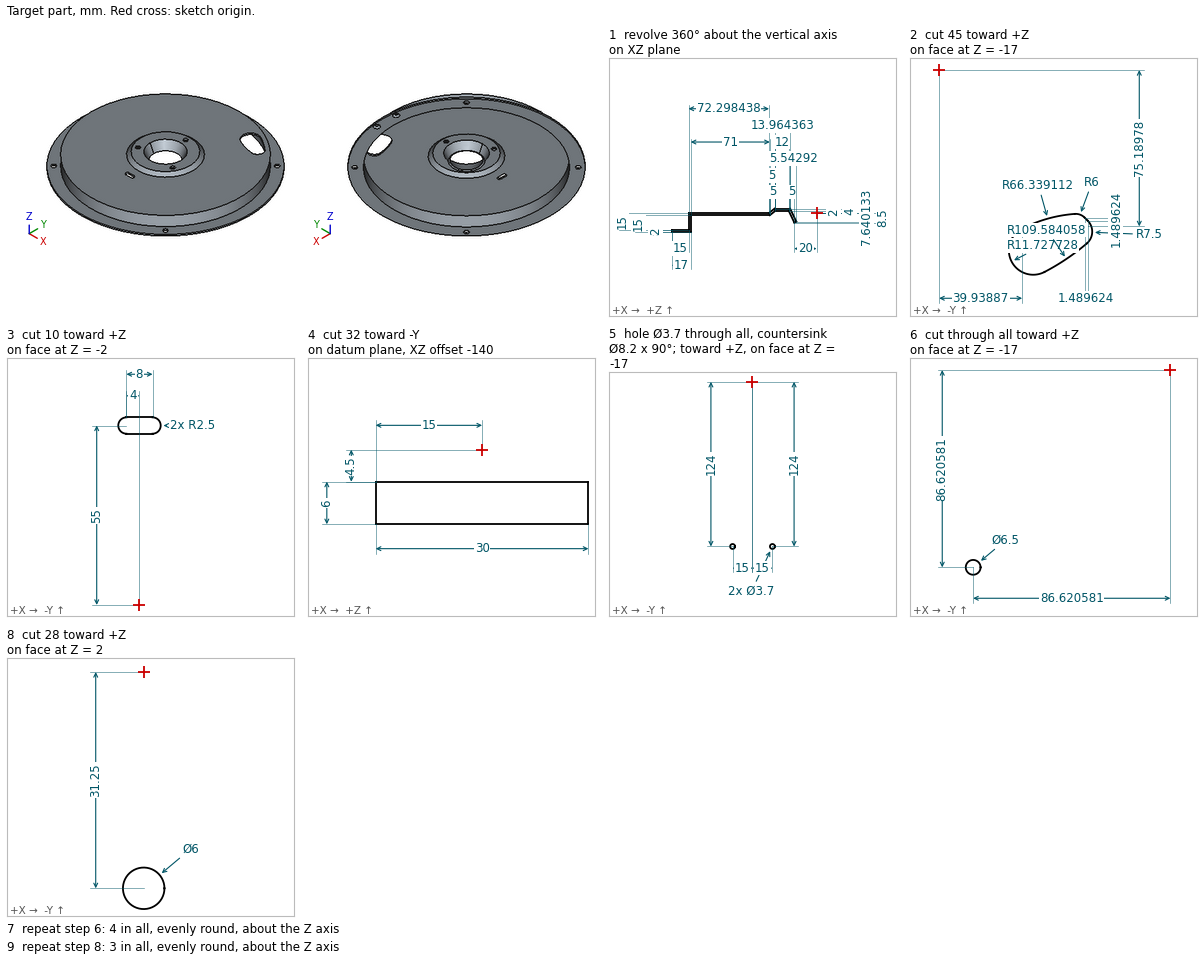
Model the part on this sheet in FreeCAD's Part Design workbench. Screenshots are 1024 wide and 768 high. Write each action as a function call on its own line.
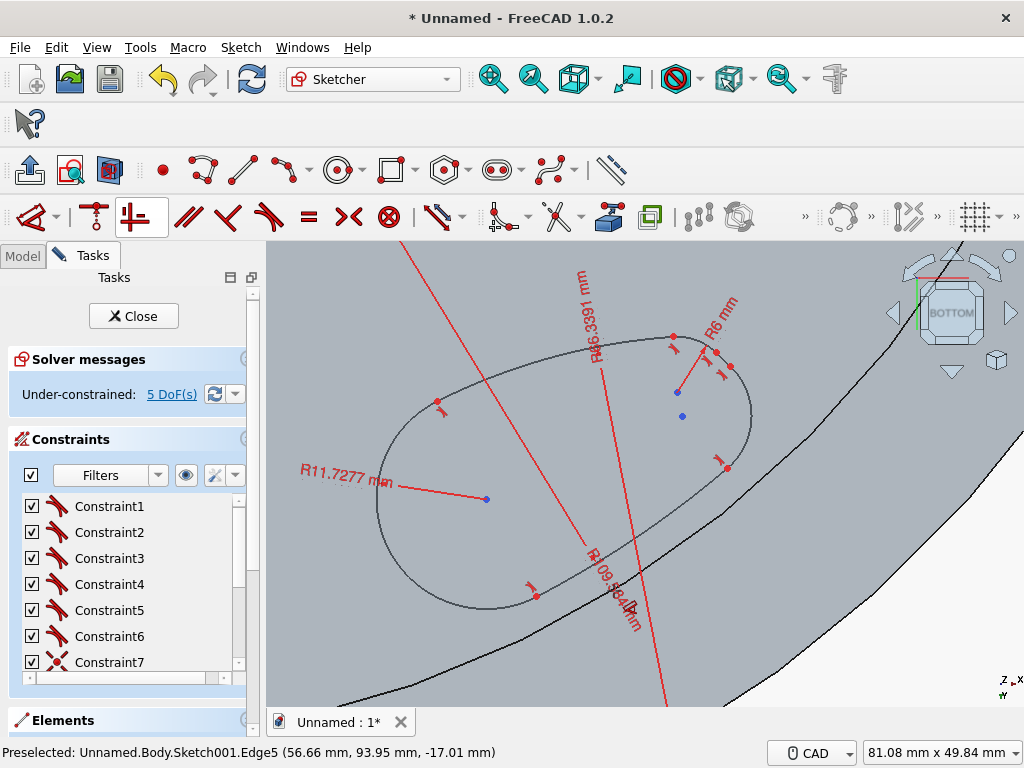
click(747, 441)
click(777, 453)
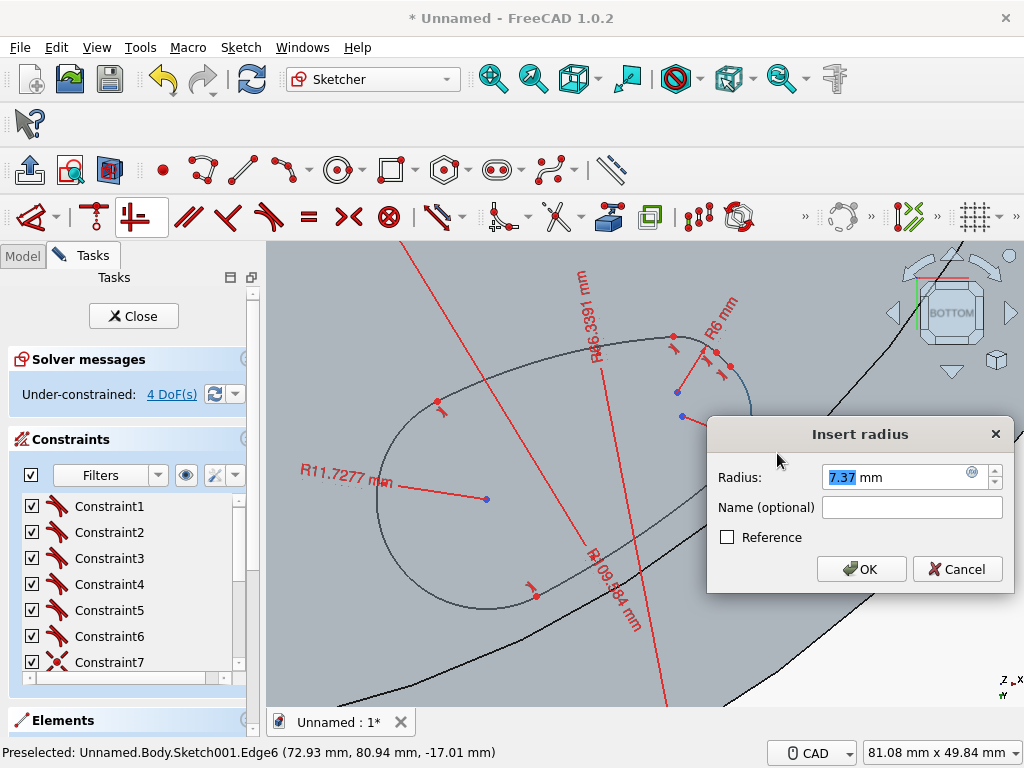
text(7.5)
key(Return)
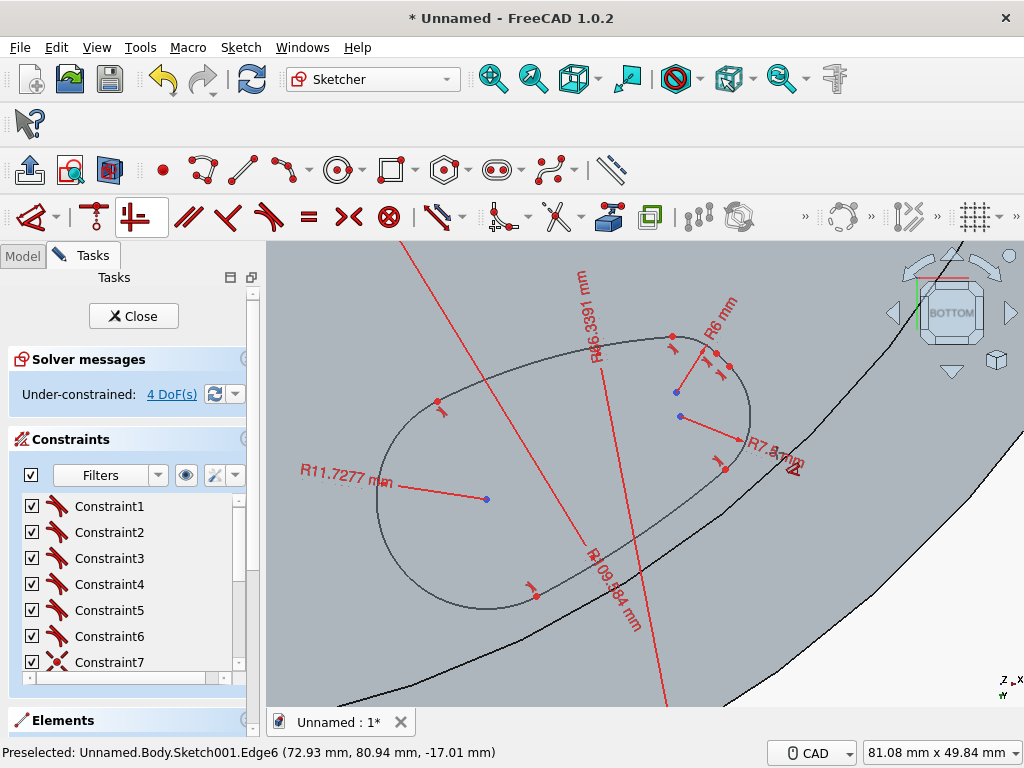
click(437, 401)
click(366, 435)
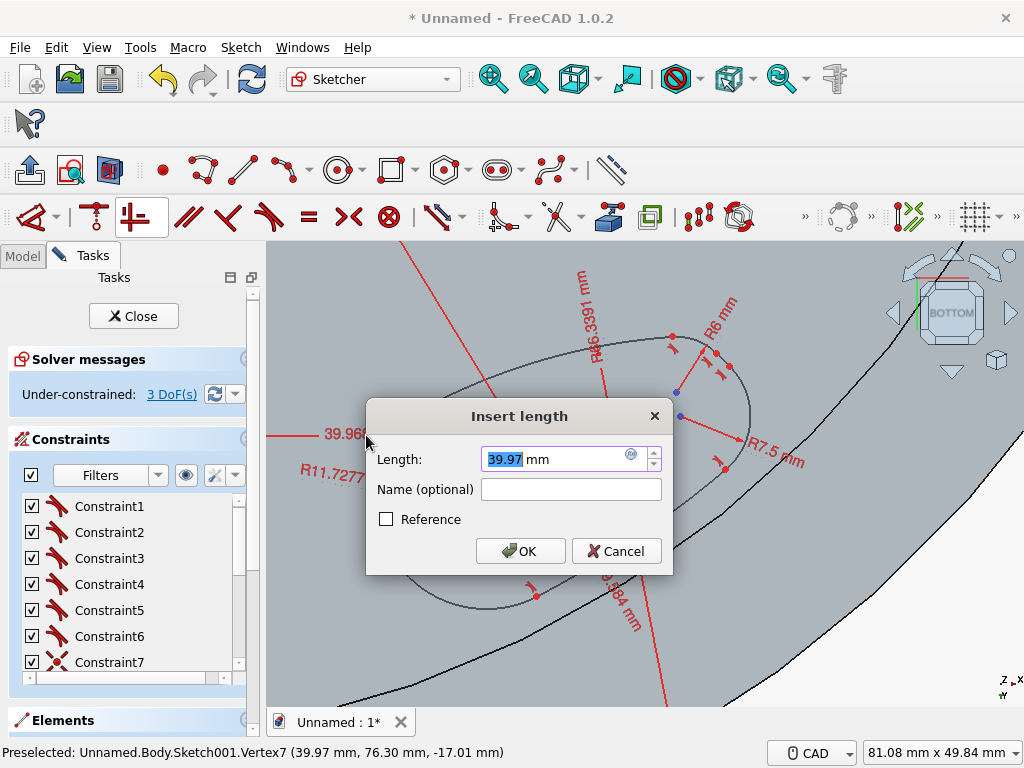
text(39.93887)
key(Return)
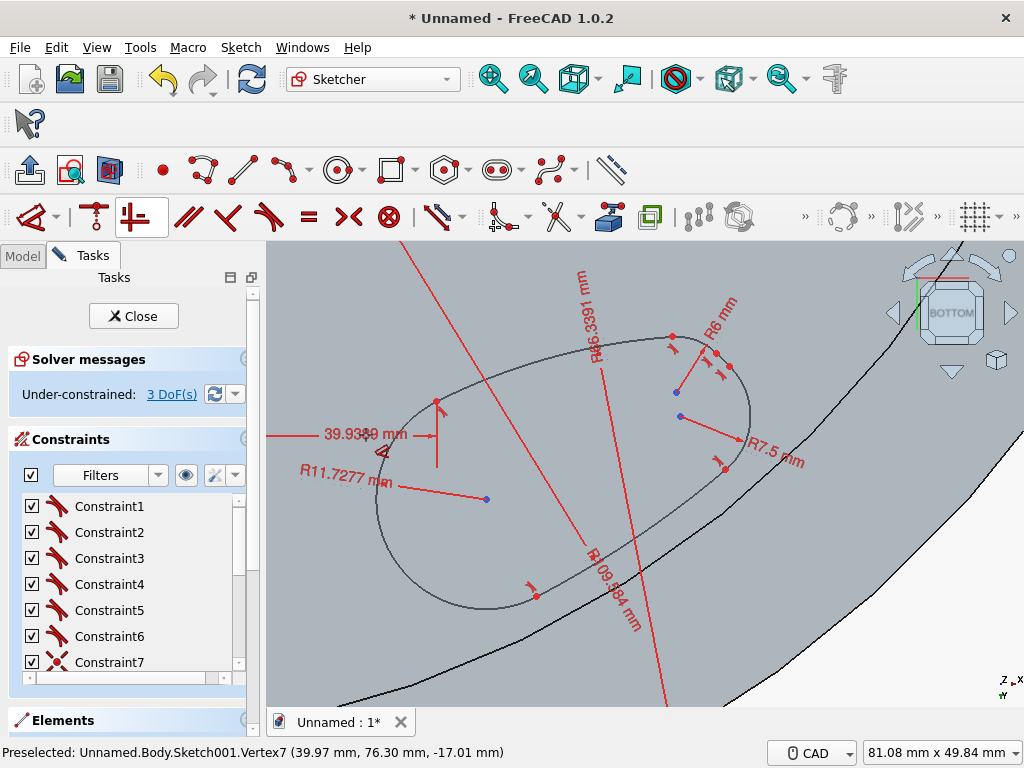
scroll(723, 360, up, 6)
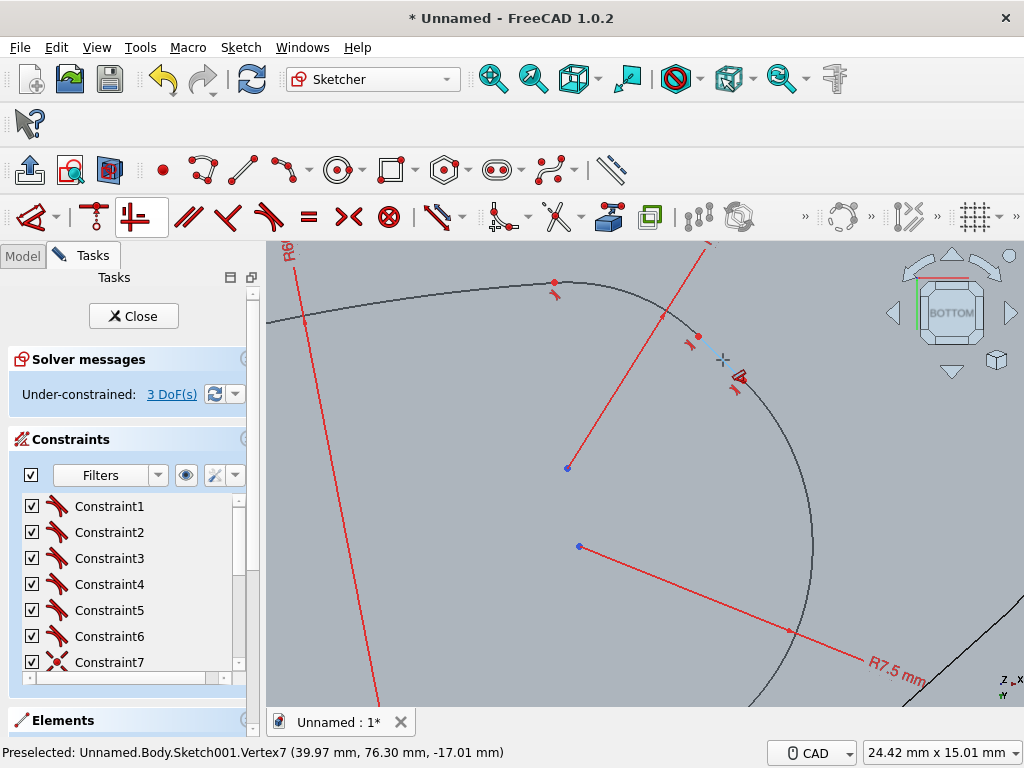
click(721, 359)
click(721, 302)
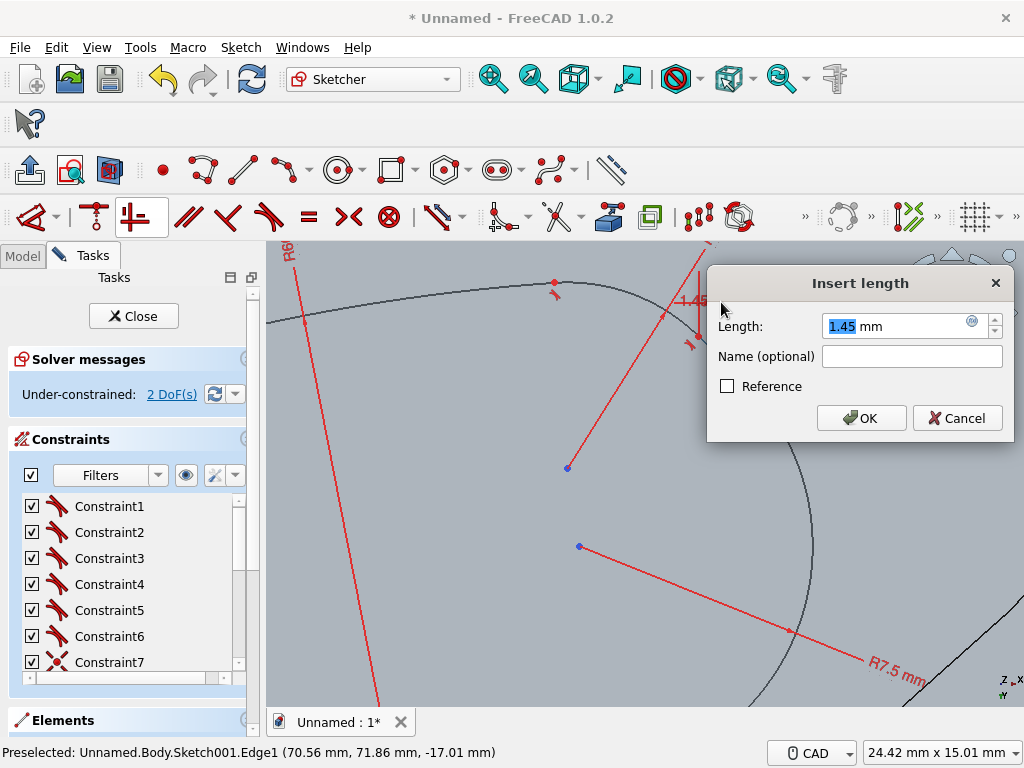
text(1.489624)
key(Return)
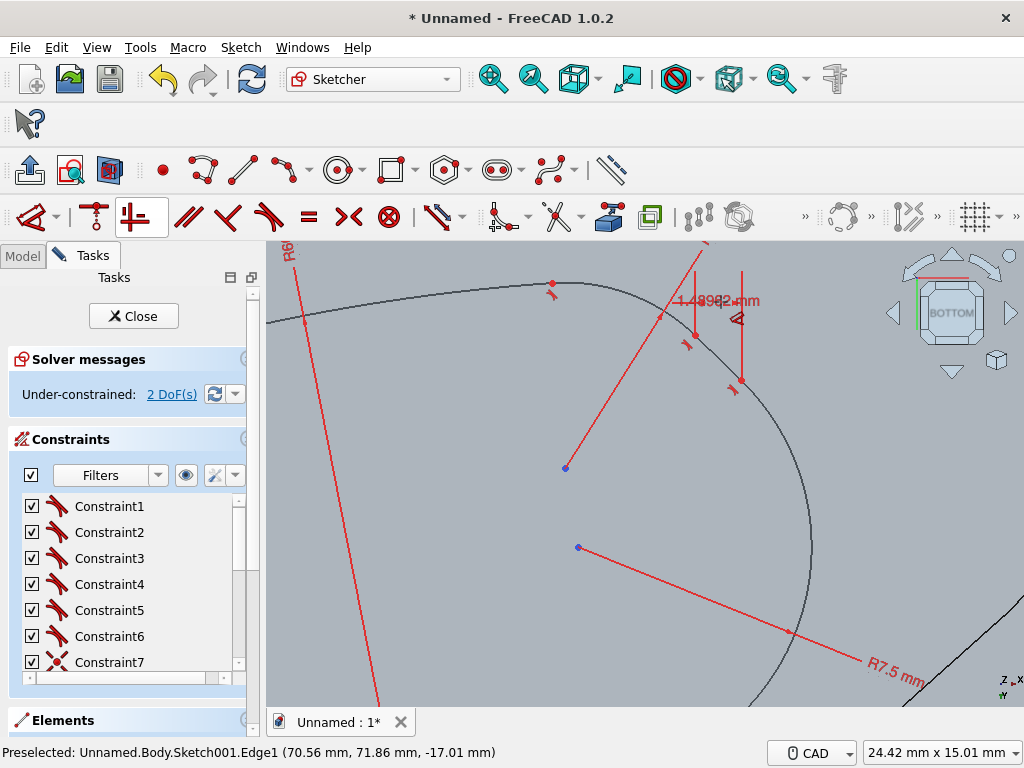
click(728, 367)
click(776, 358)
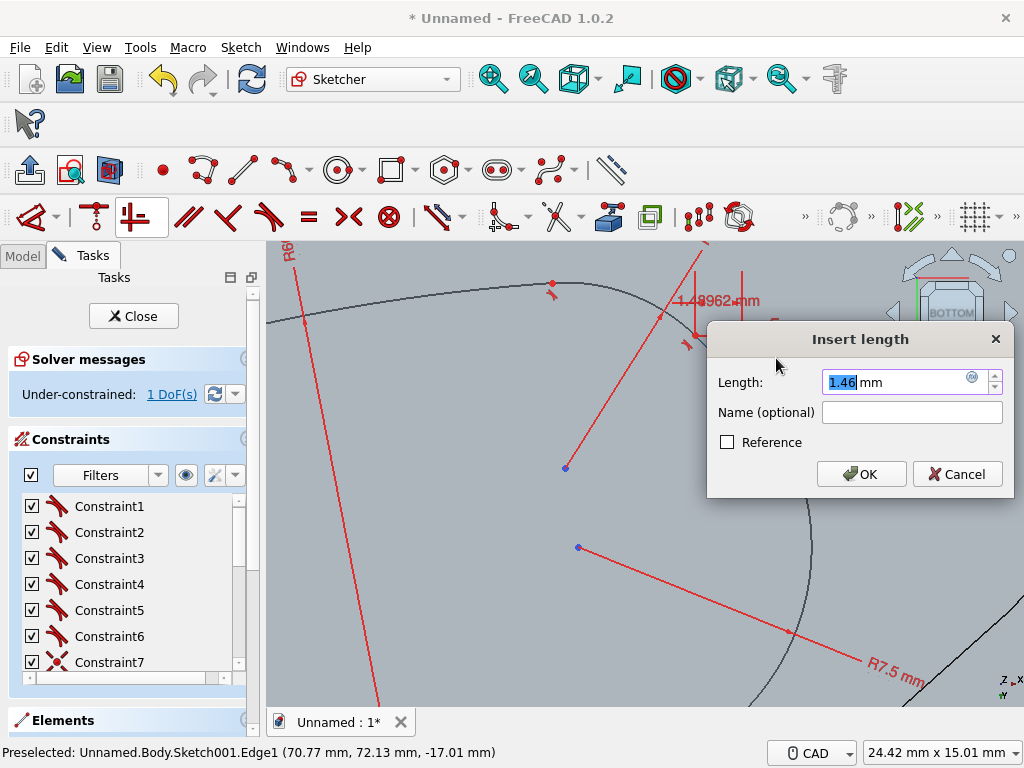
text(1.489624)
key(Return)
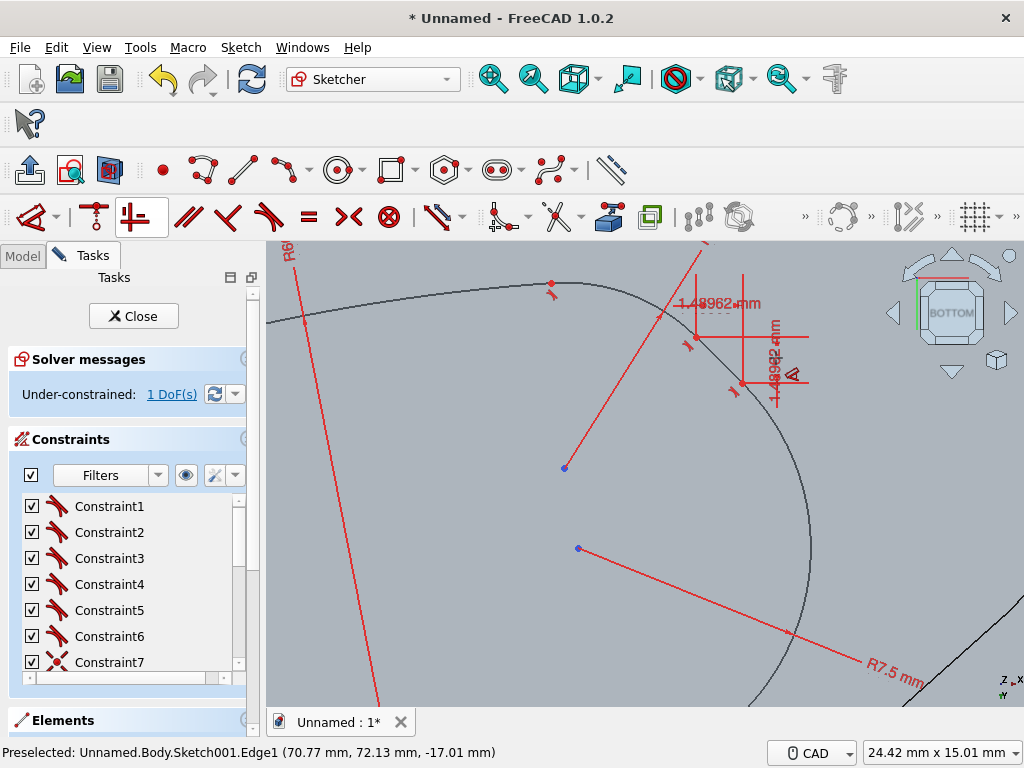
click(565, 469)
click(599, 369)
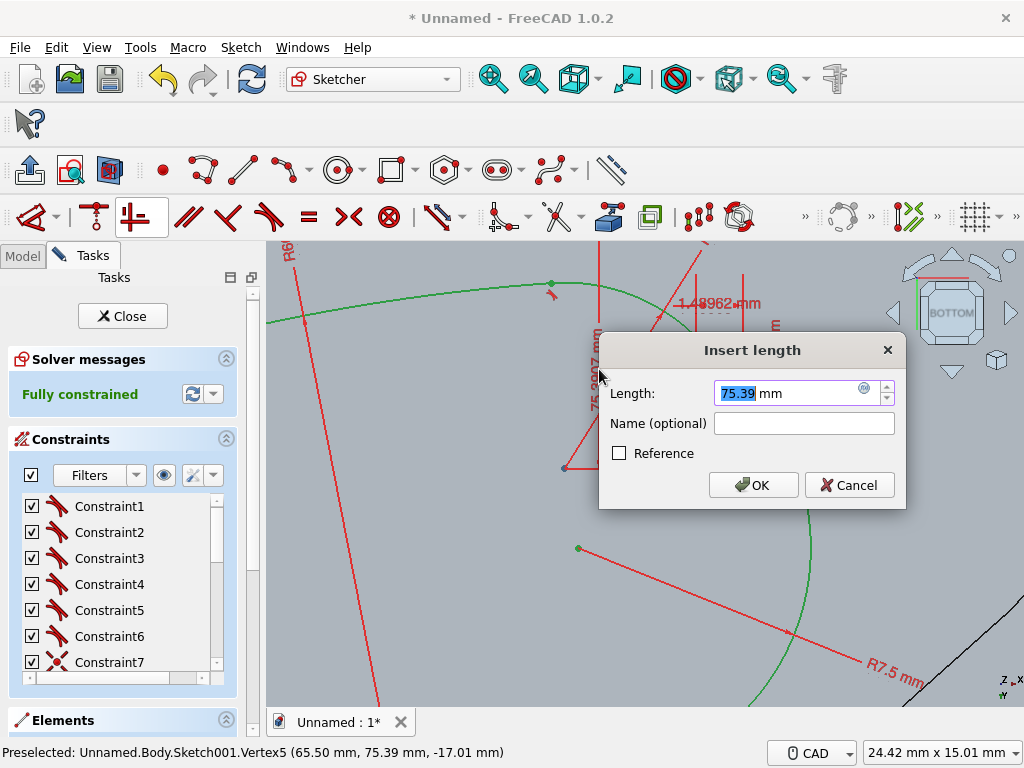
text(75.18978)
key(Return)
key(Escape)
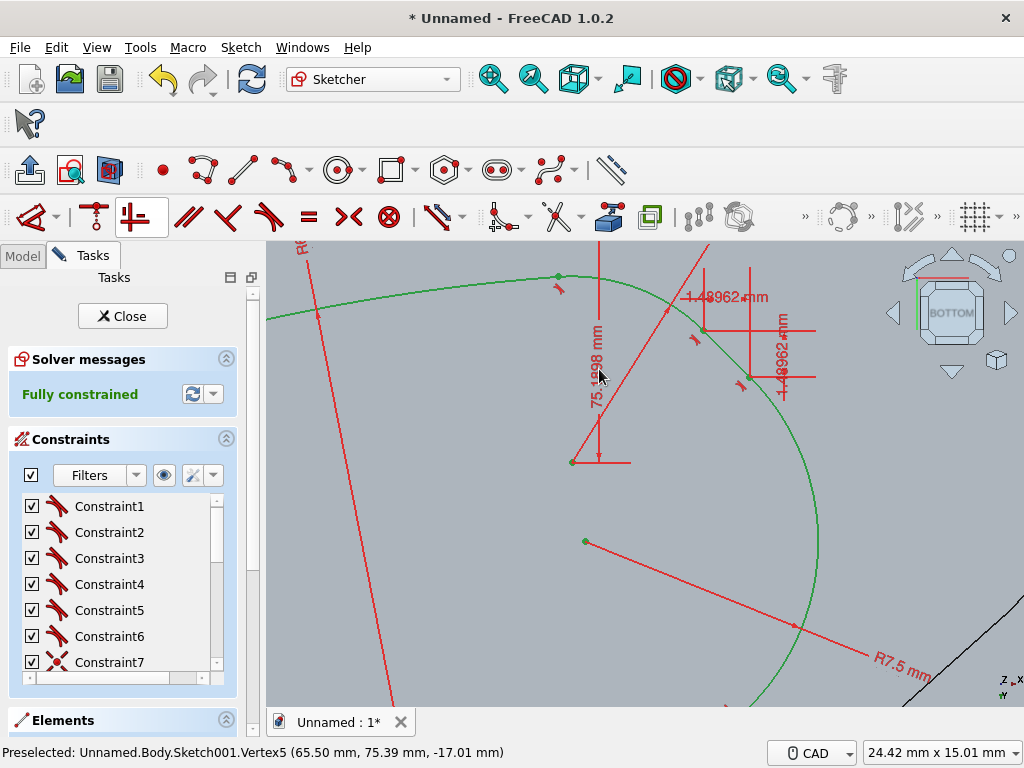
click(123, 316)